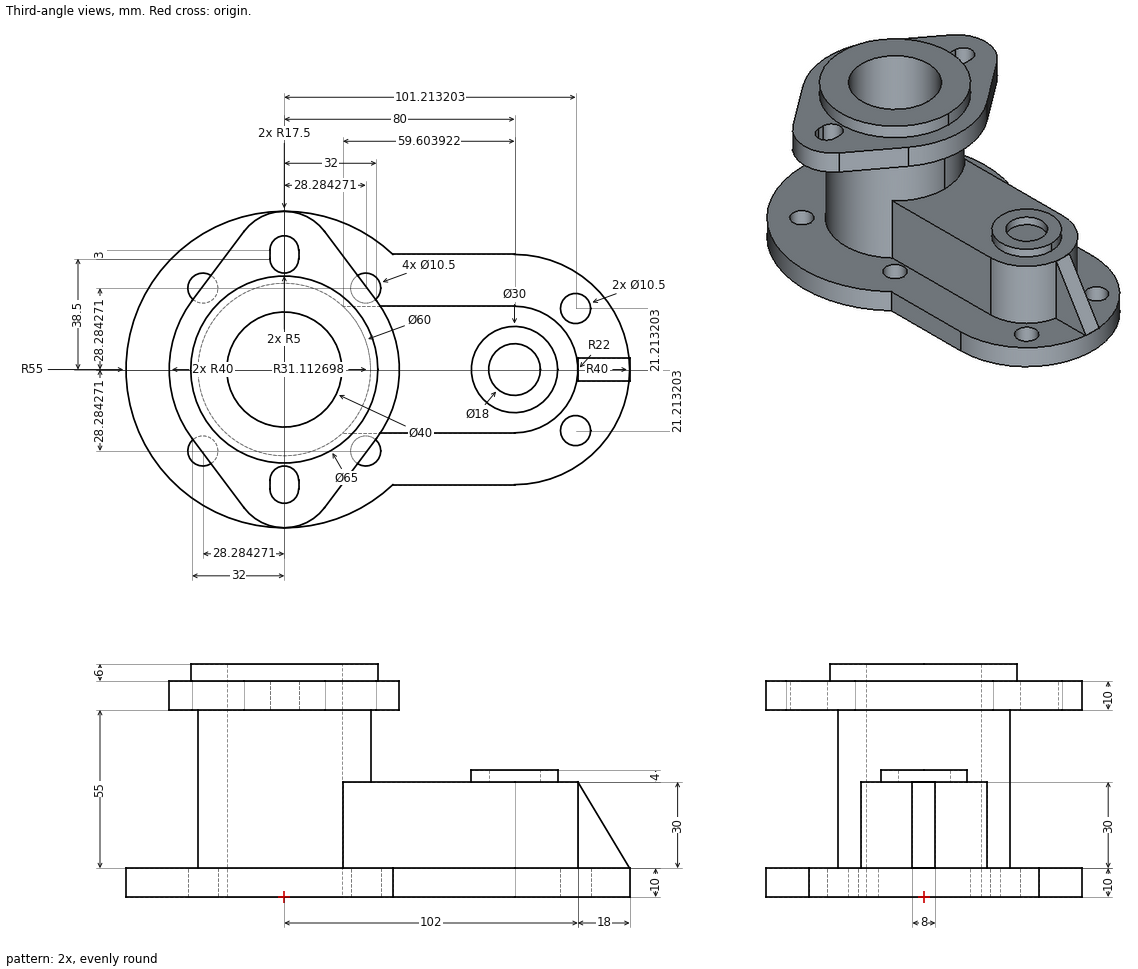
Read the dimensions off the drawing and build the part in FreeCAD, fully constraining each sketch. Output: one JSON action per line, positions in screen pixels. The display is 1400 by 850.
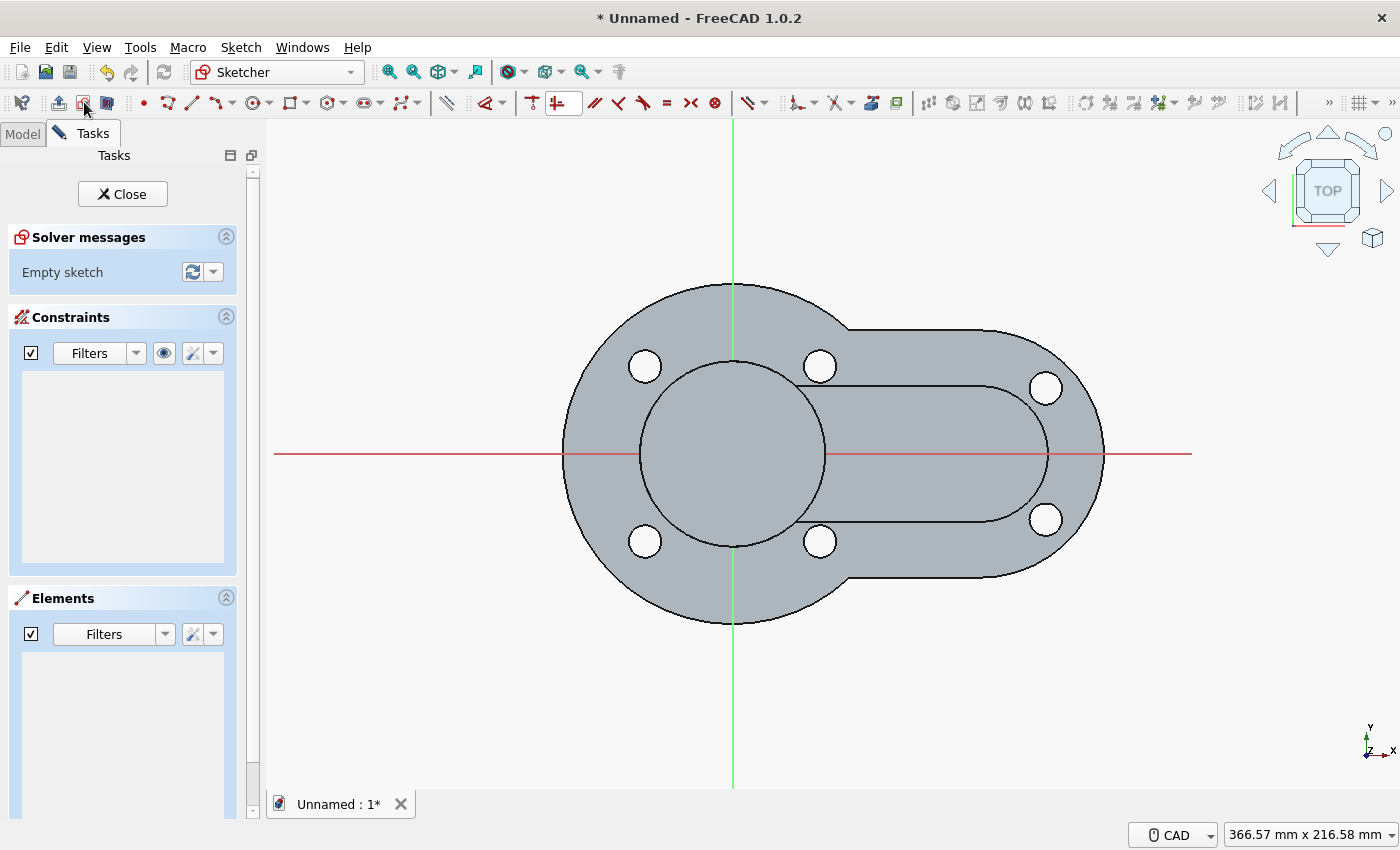
{"action": "key", "text": "q s"}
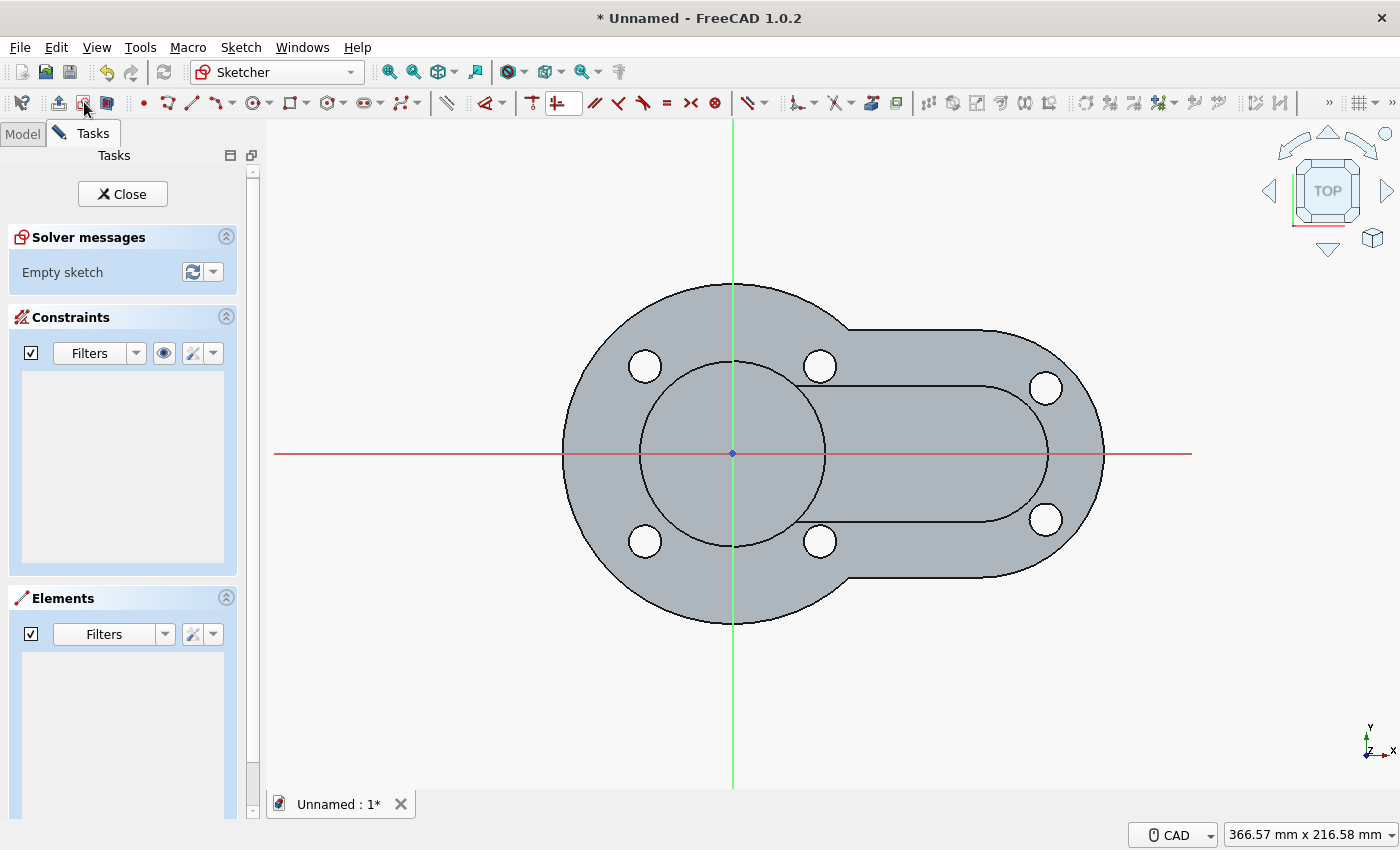
{"action": "scroll", "coordinate": [1035, 454], "scroll_direction": "up", "scroll_amount": 8}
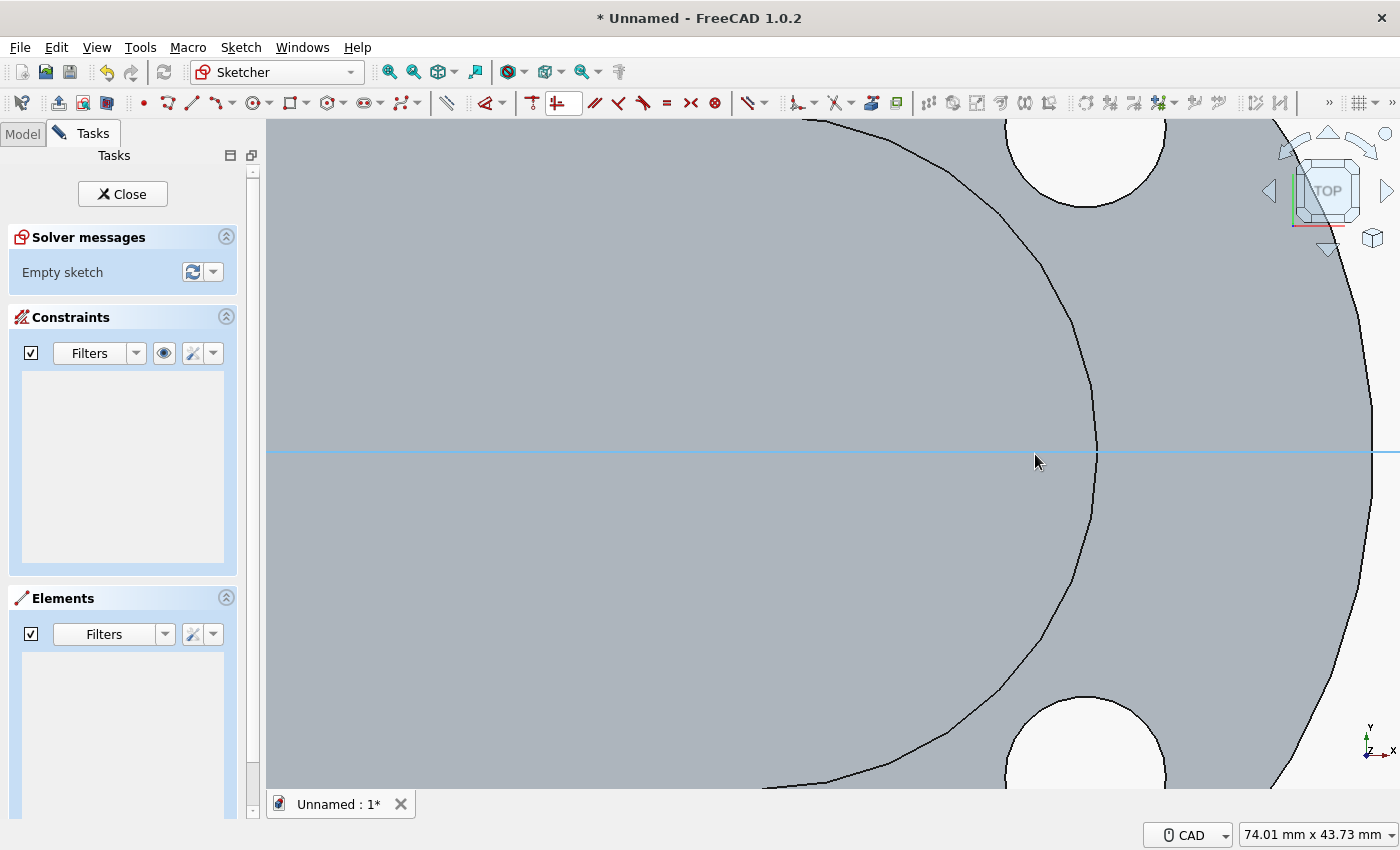
{"action": "left_click", "coordinate": [254, 104]}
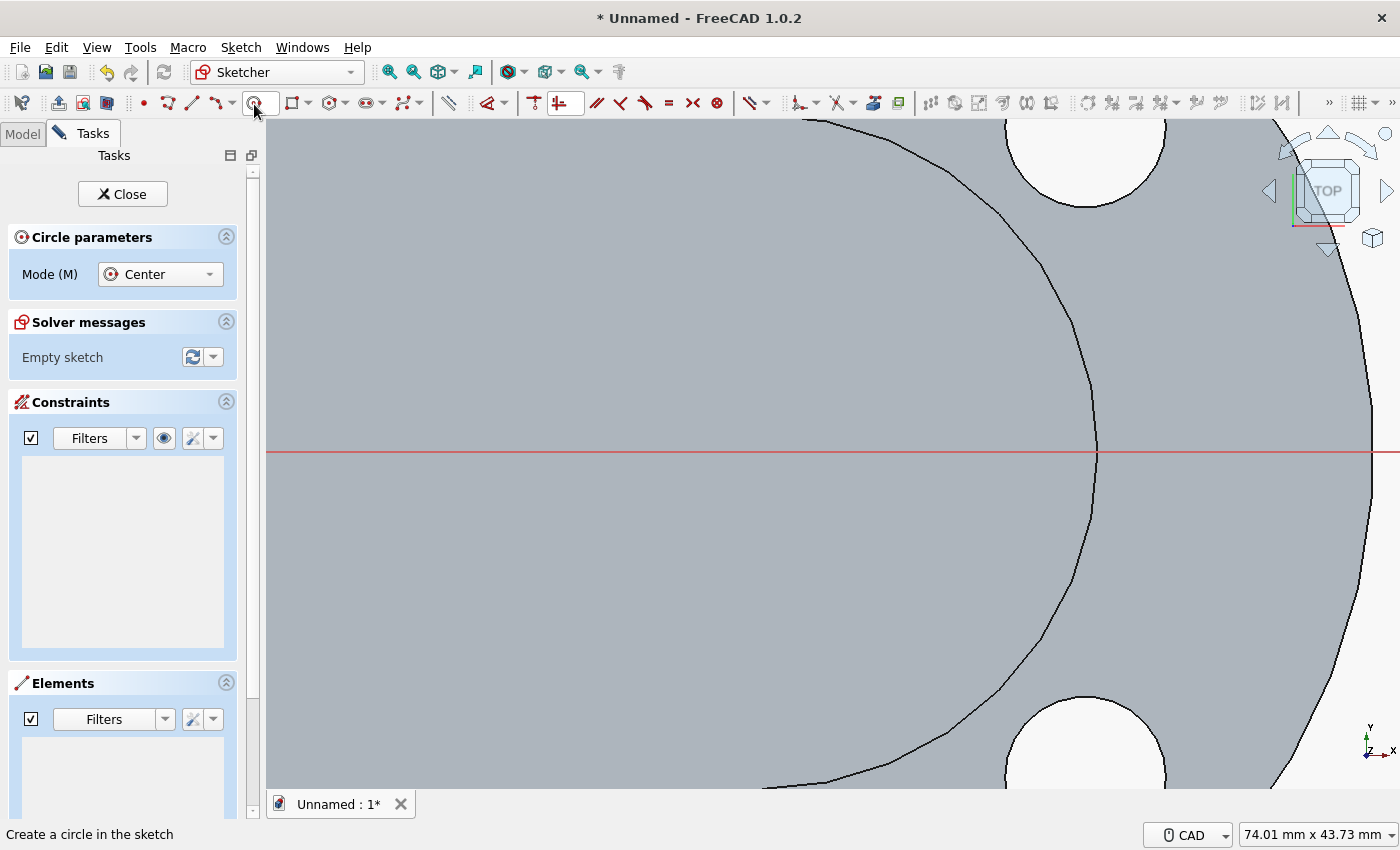
{"action": "left_click", "coordinate": [760, 452]}
{"action": "mouse_move", "coordinate": [923, 290]}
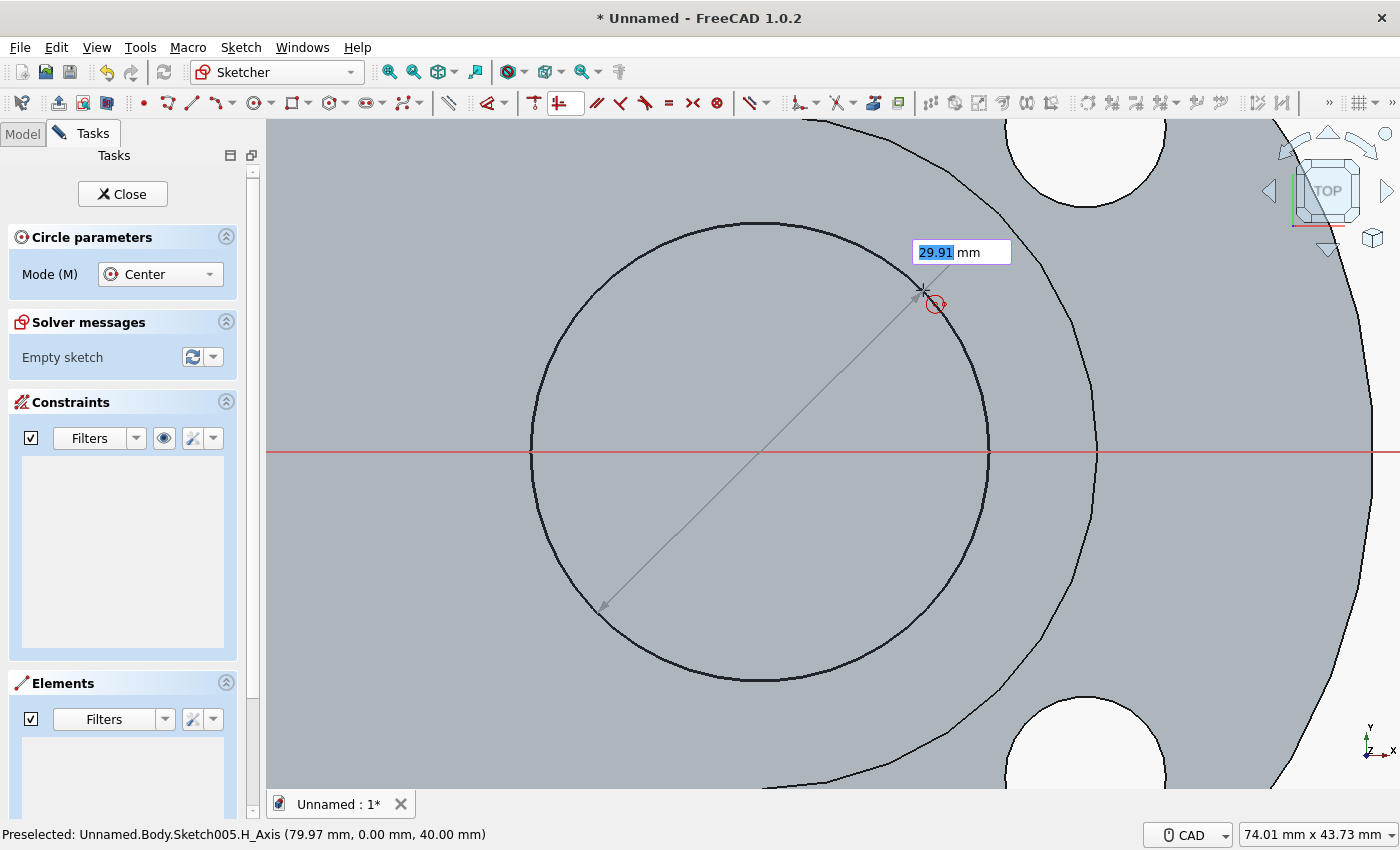
{"action": "type", "text": "30"}
{"action": "key", "text": "Return"}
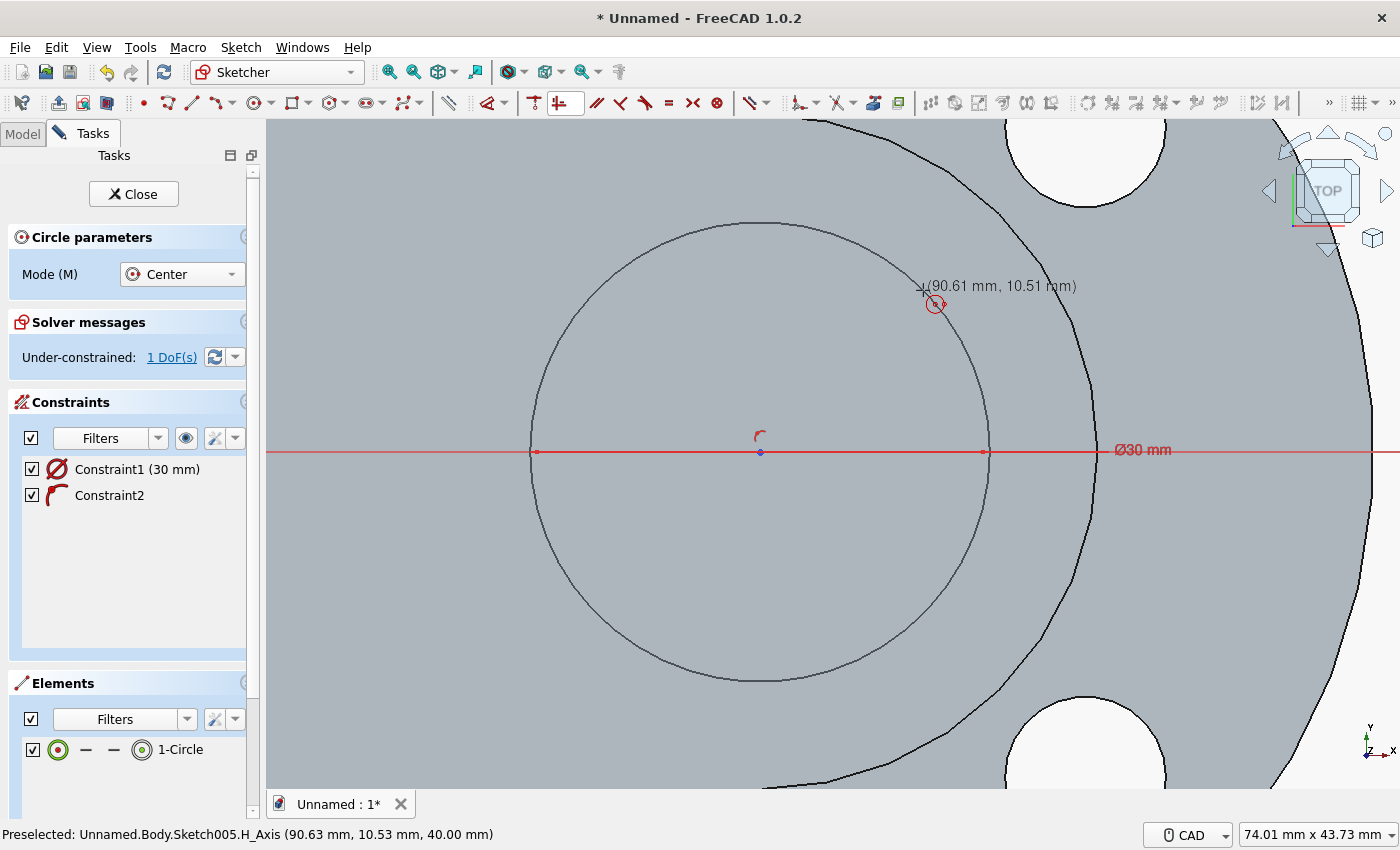
{"action": "left_click", "coordinate": [760, 452]}
{"action": "mouse_move", "coordinate": [858, 355]}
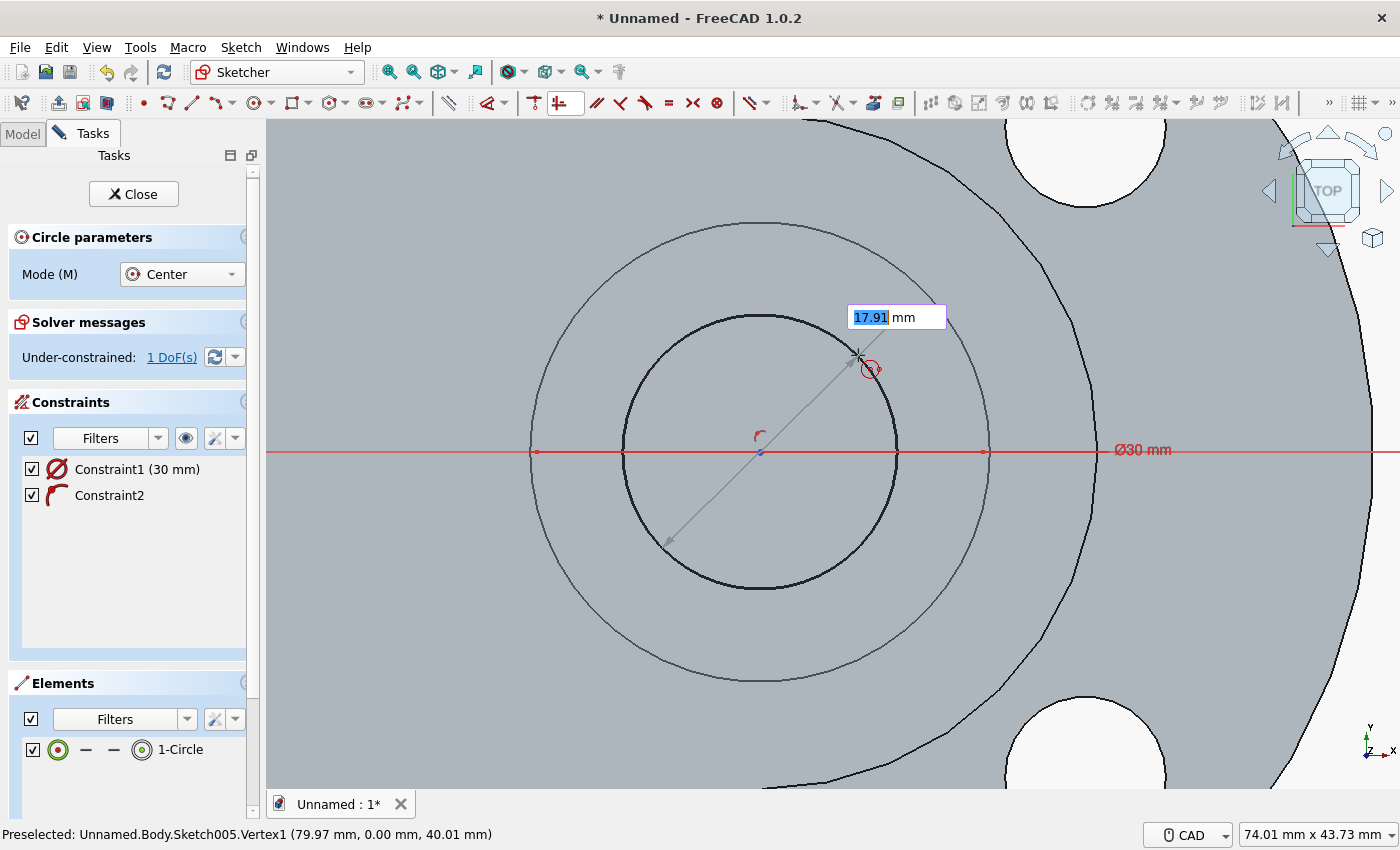
{"action": "type", "text": "18"}
{"action": "key", "text": "Return"}
{"action": "key", "text": "Escape"}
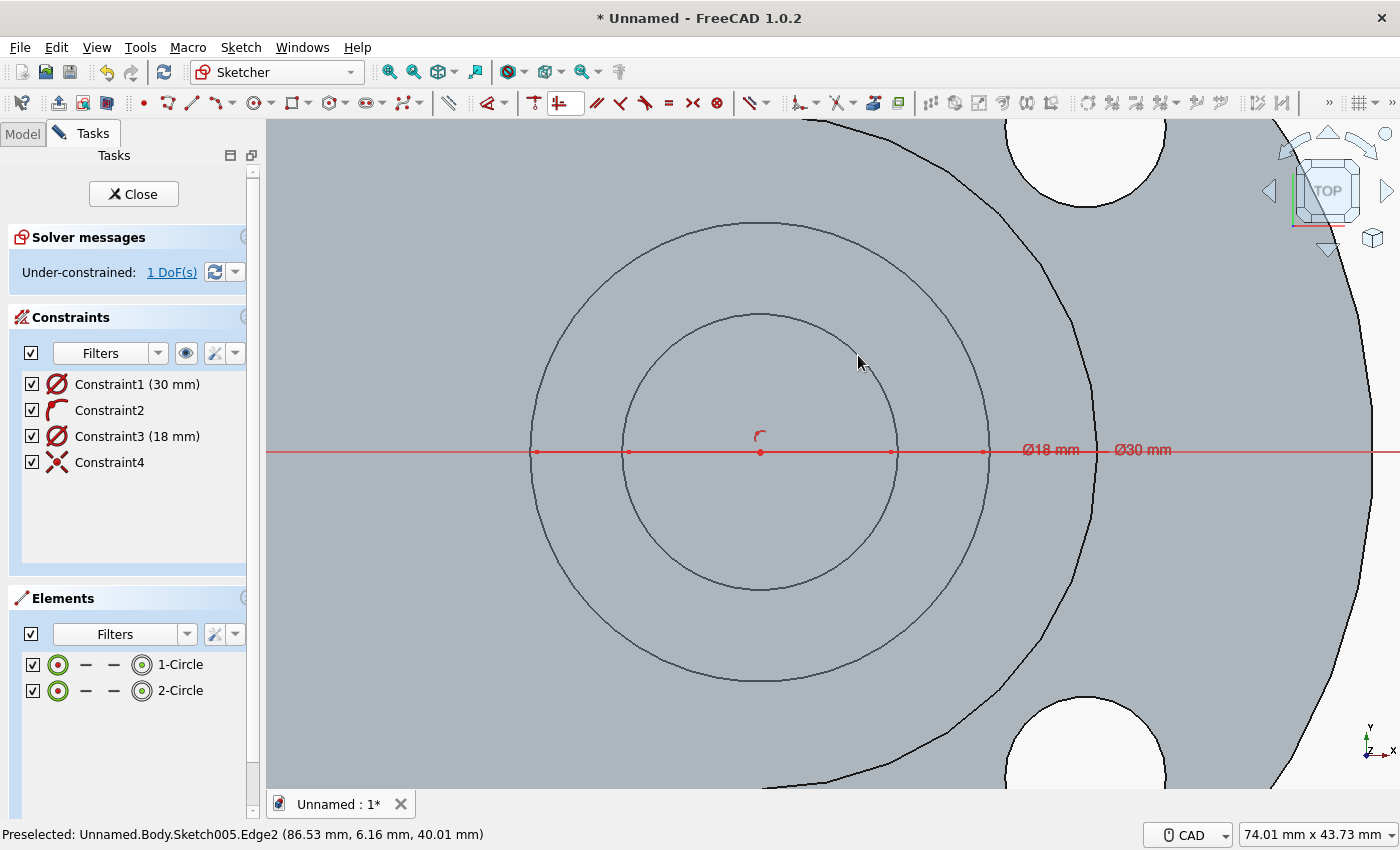
{"action": "left_click", "coordinate": [488, 104]}